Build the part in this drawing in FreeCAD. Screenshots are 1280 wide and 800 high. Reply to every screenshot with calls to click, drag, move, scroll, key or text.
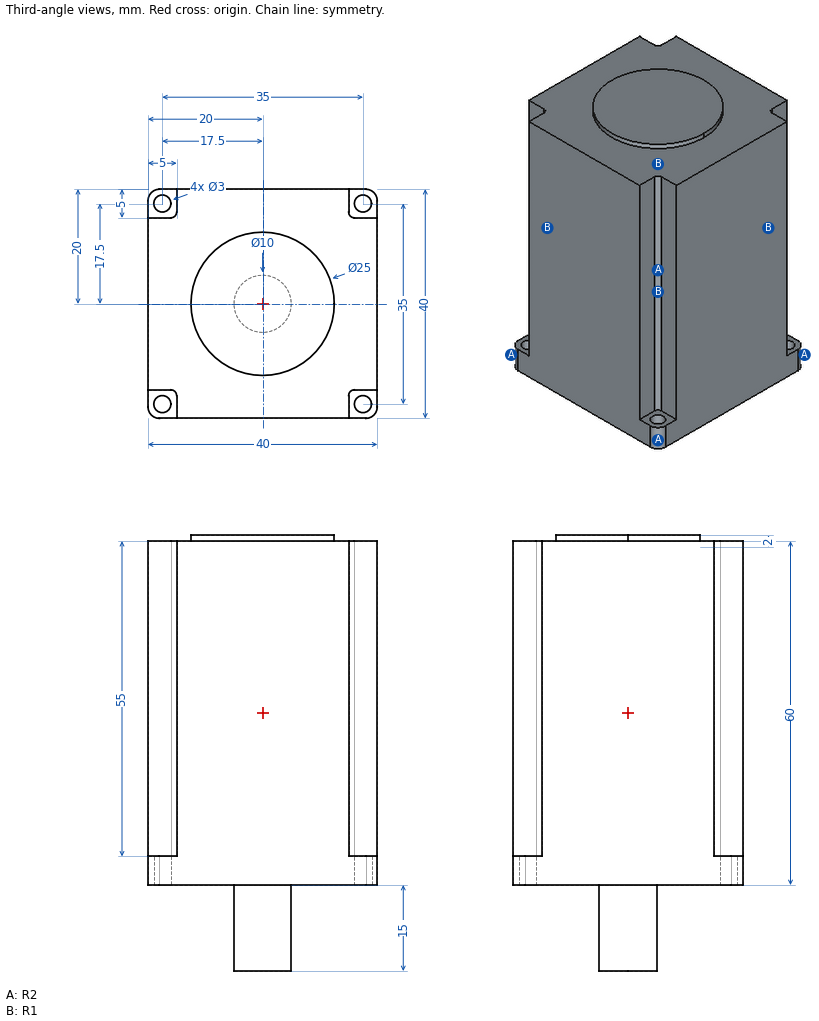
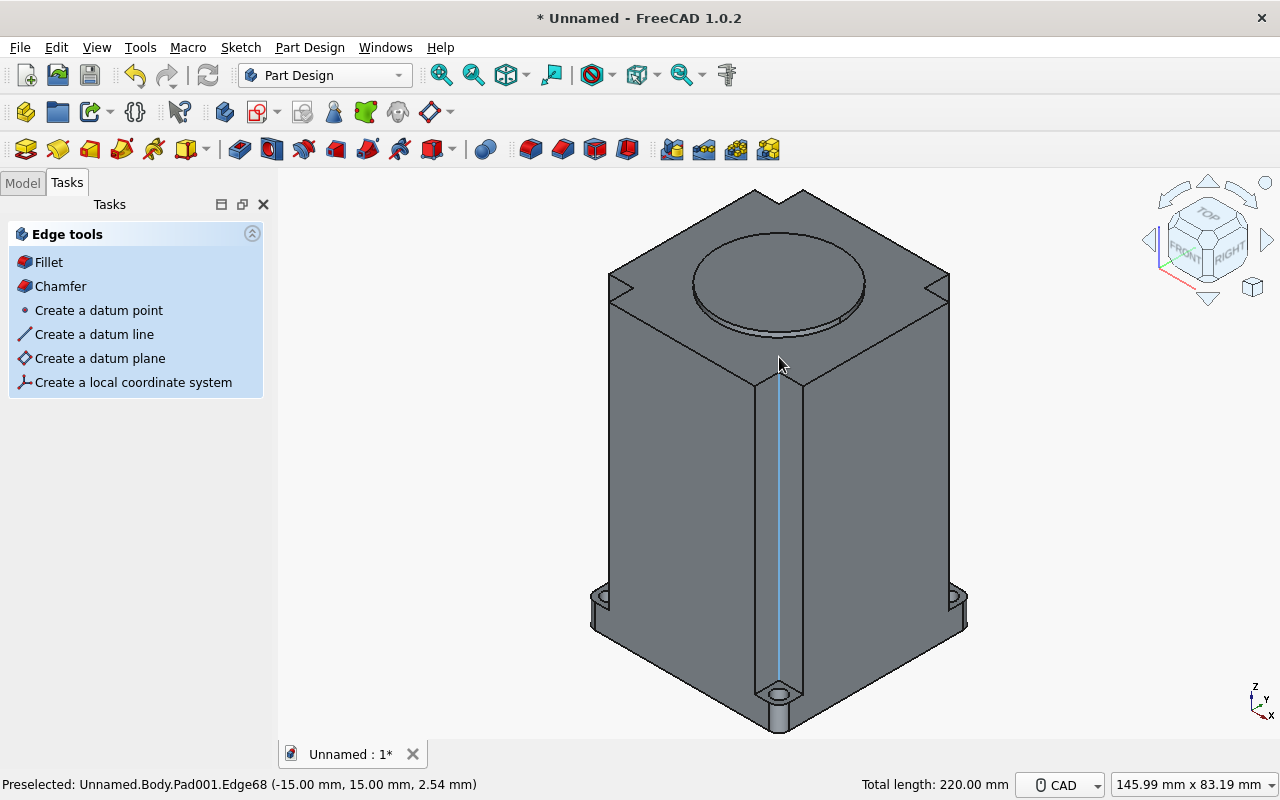
click(532, 150)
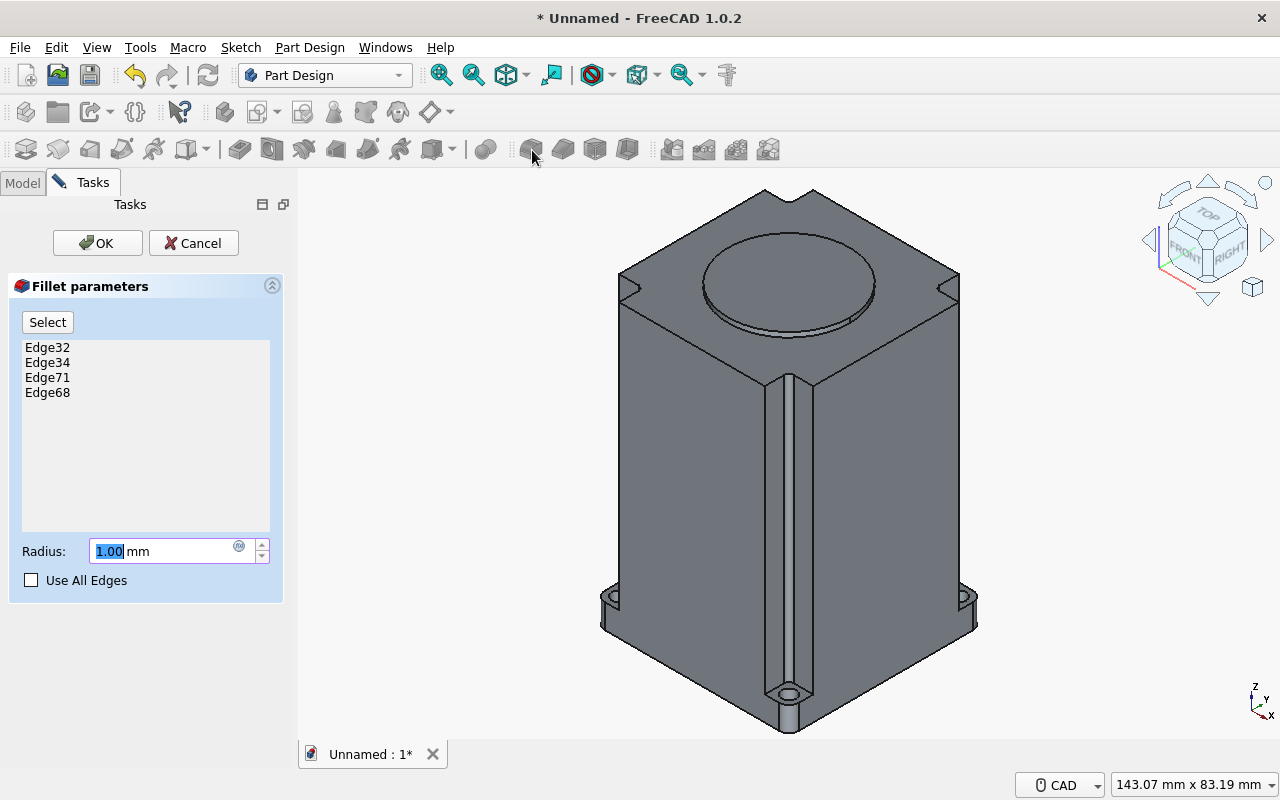
text(1)
key(Tab)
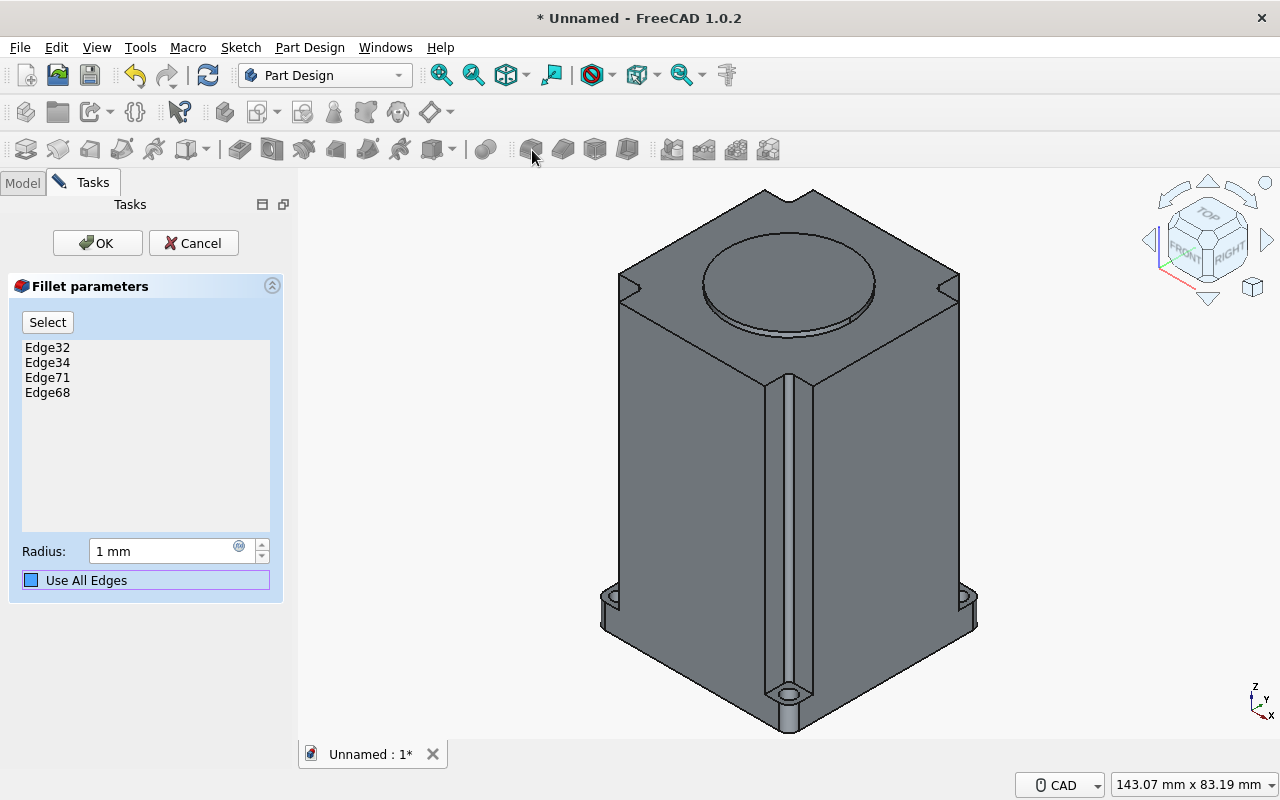
click(98, 243)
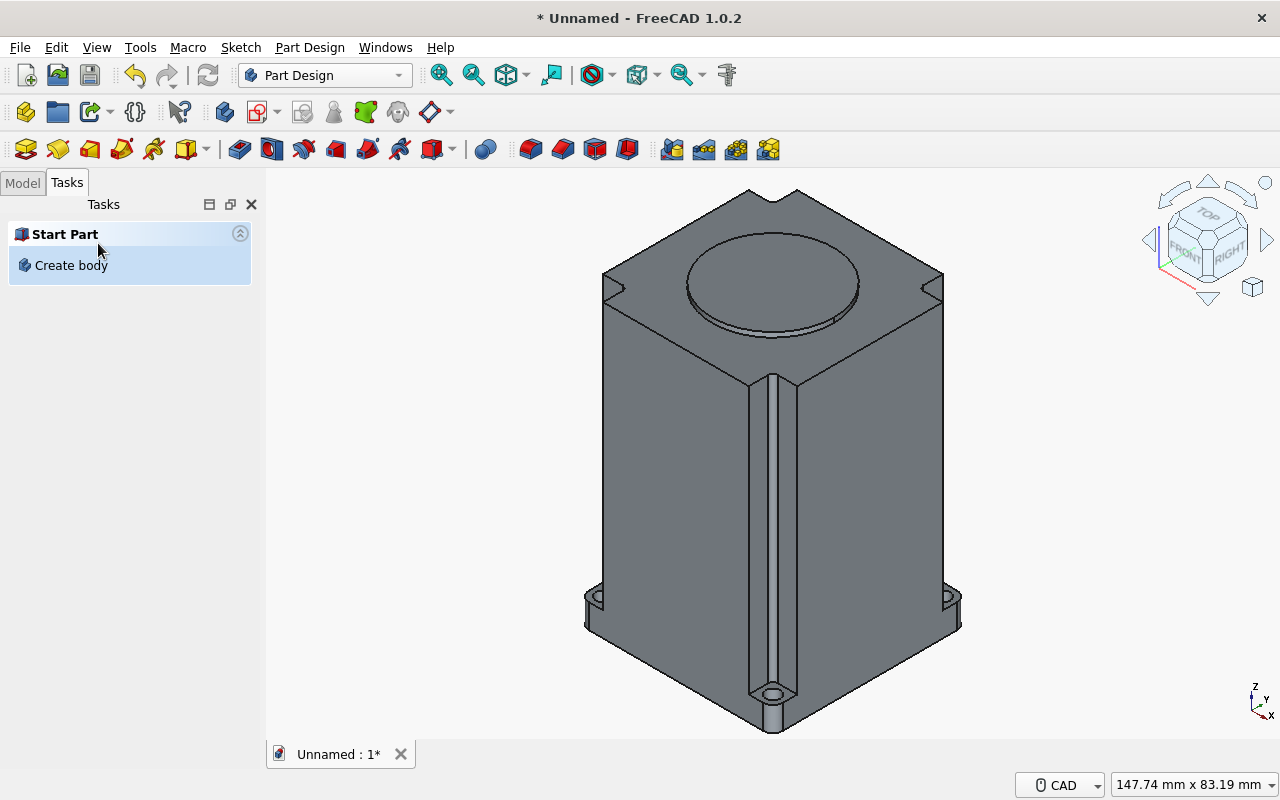
key(5)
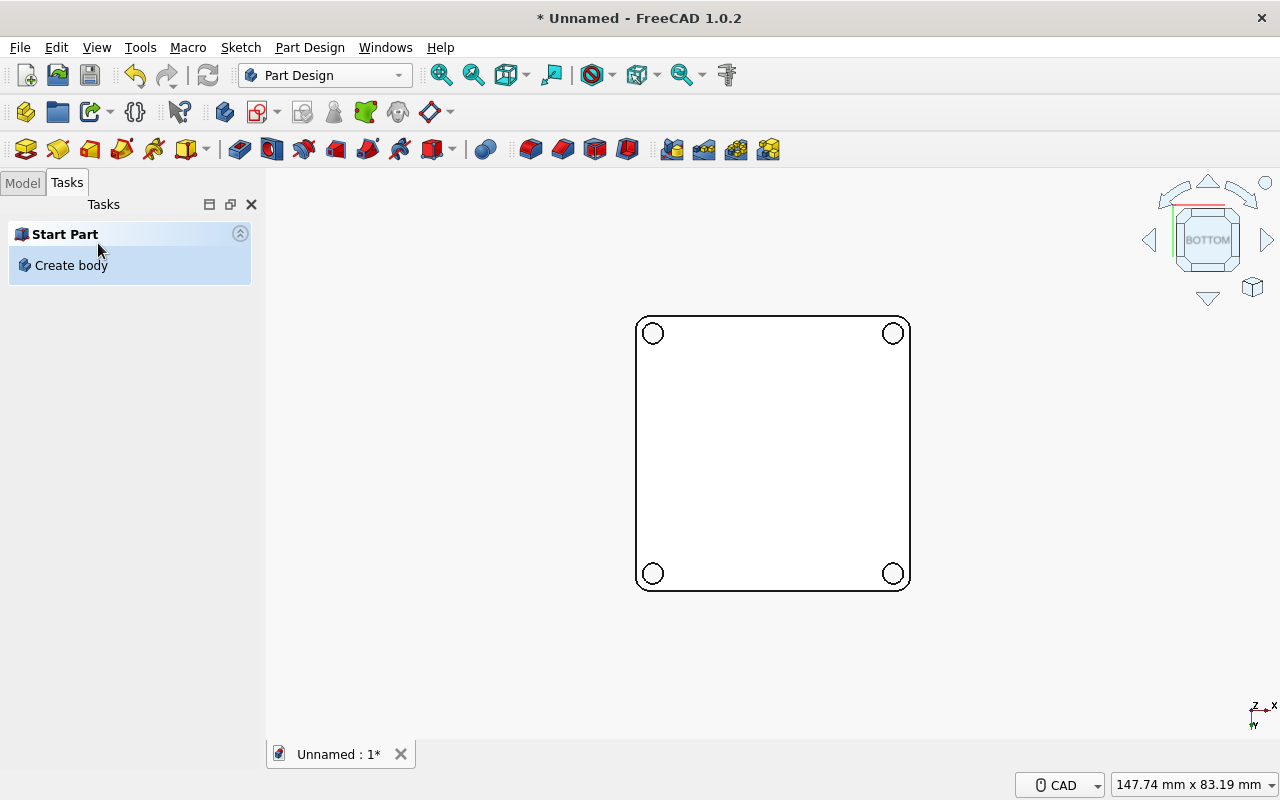
click(773, 452)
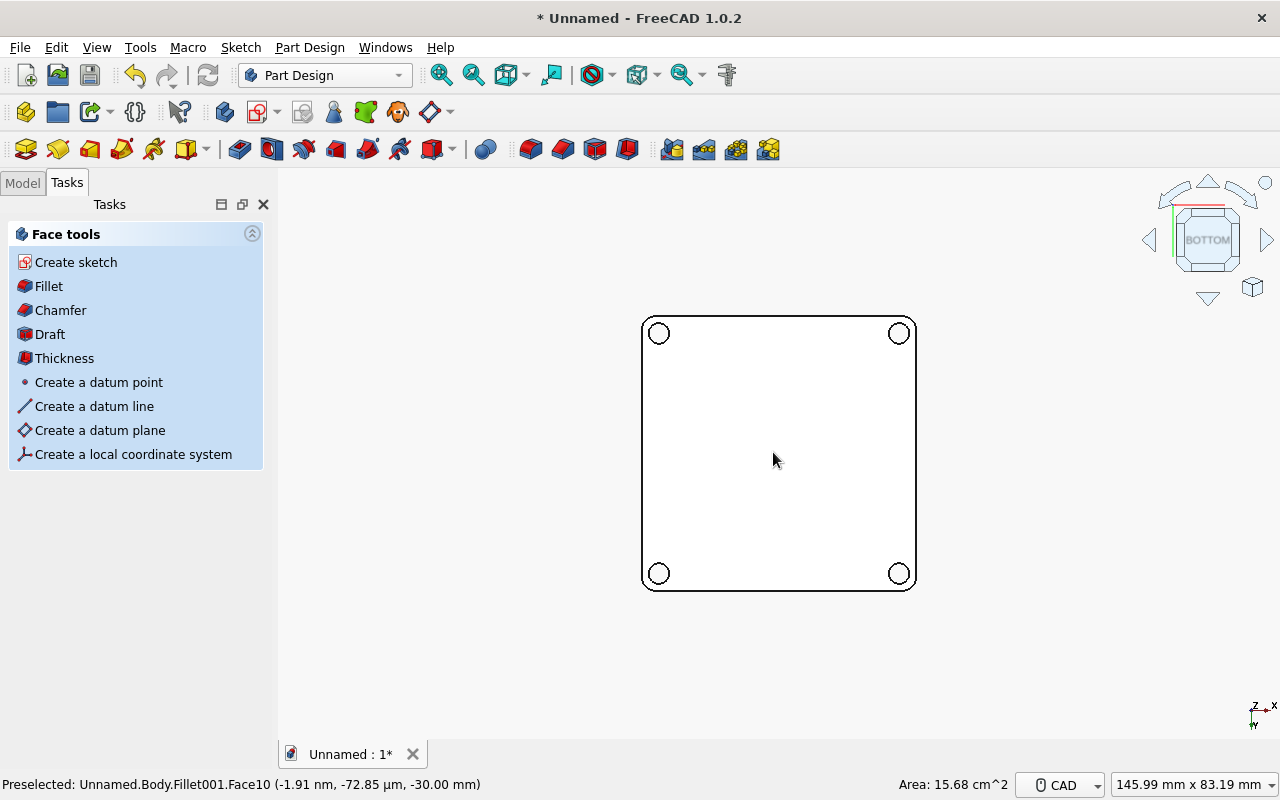
click(258, 112)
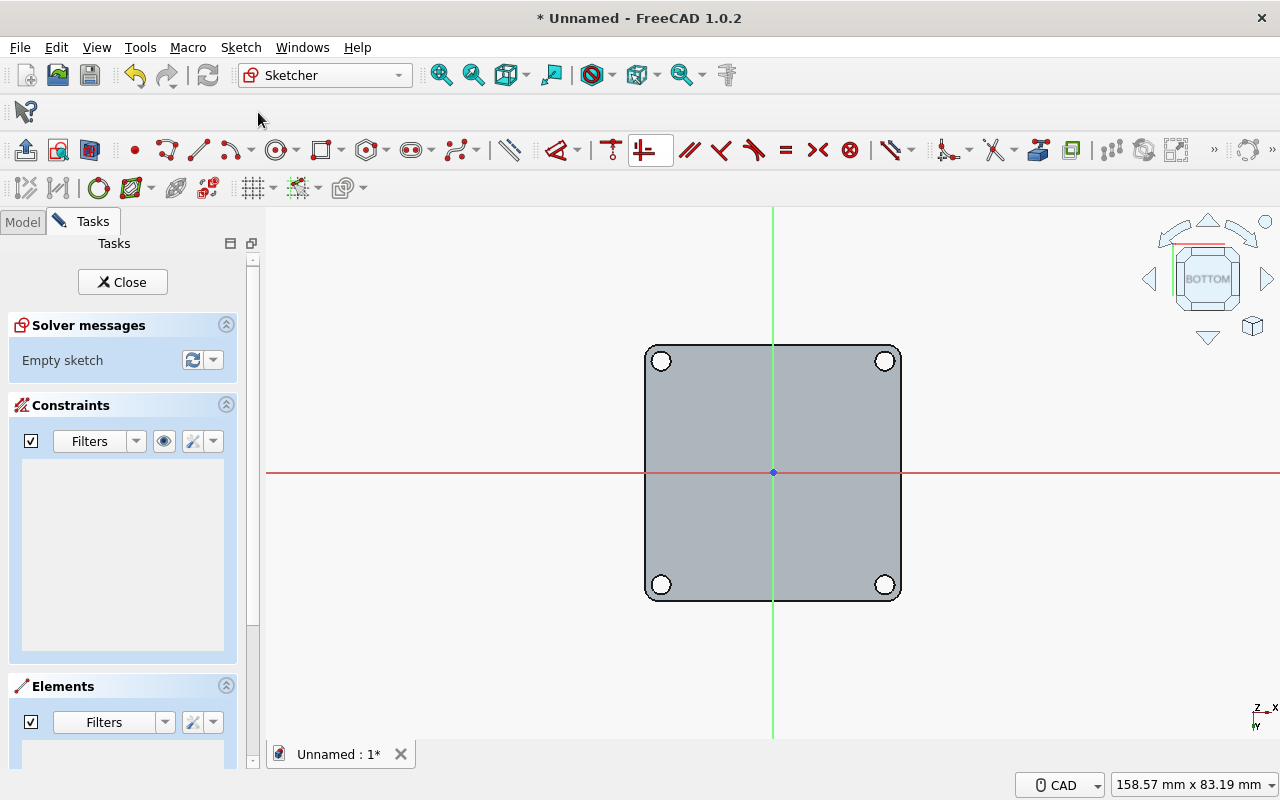
scroll(790, 473, up, 8)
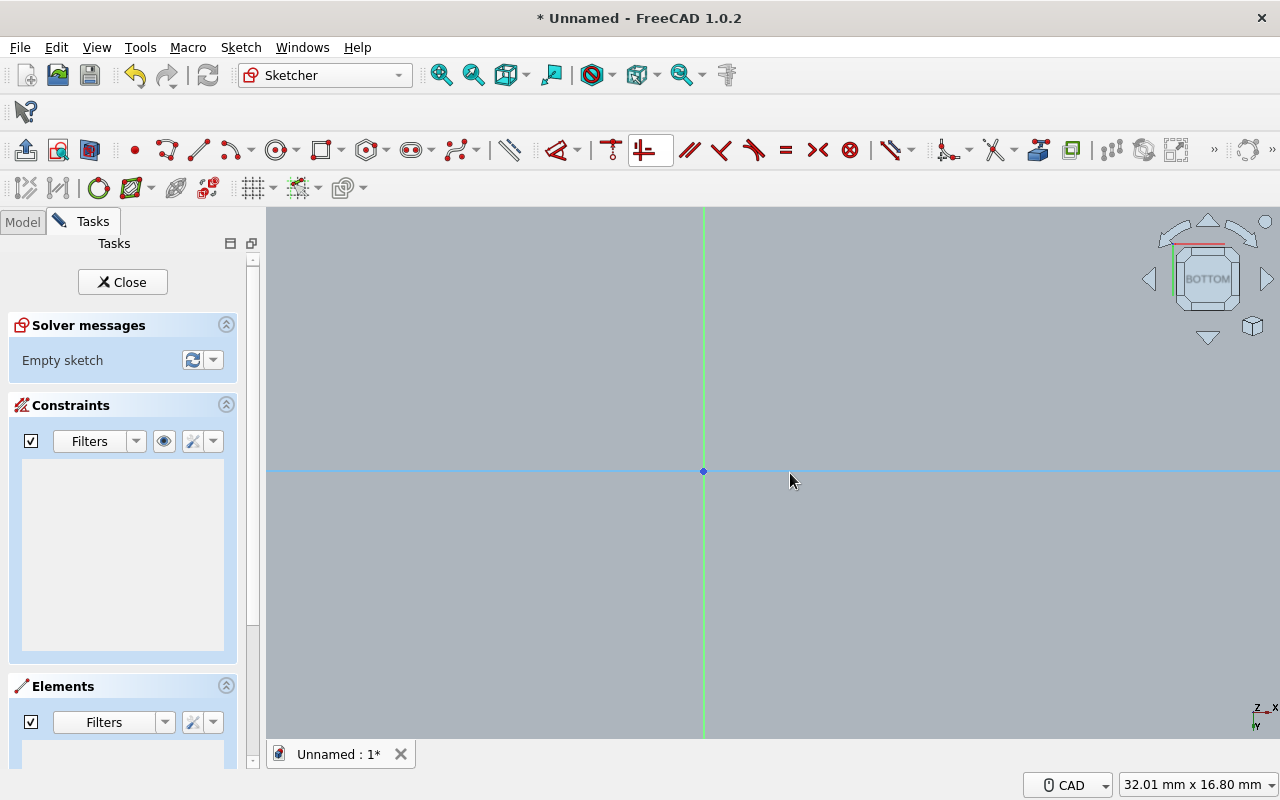
click(276, 150)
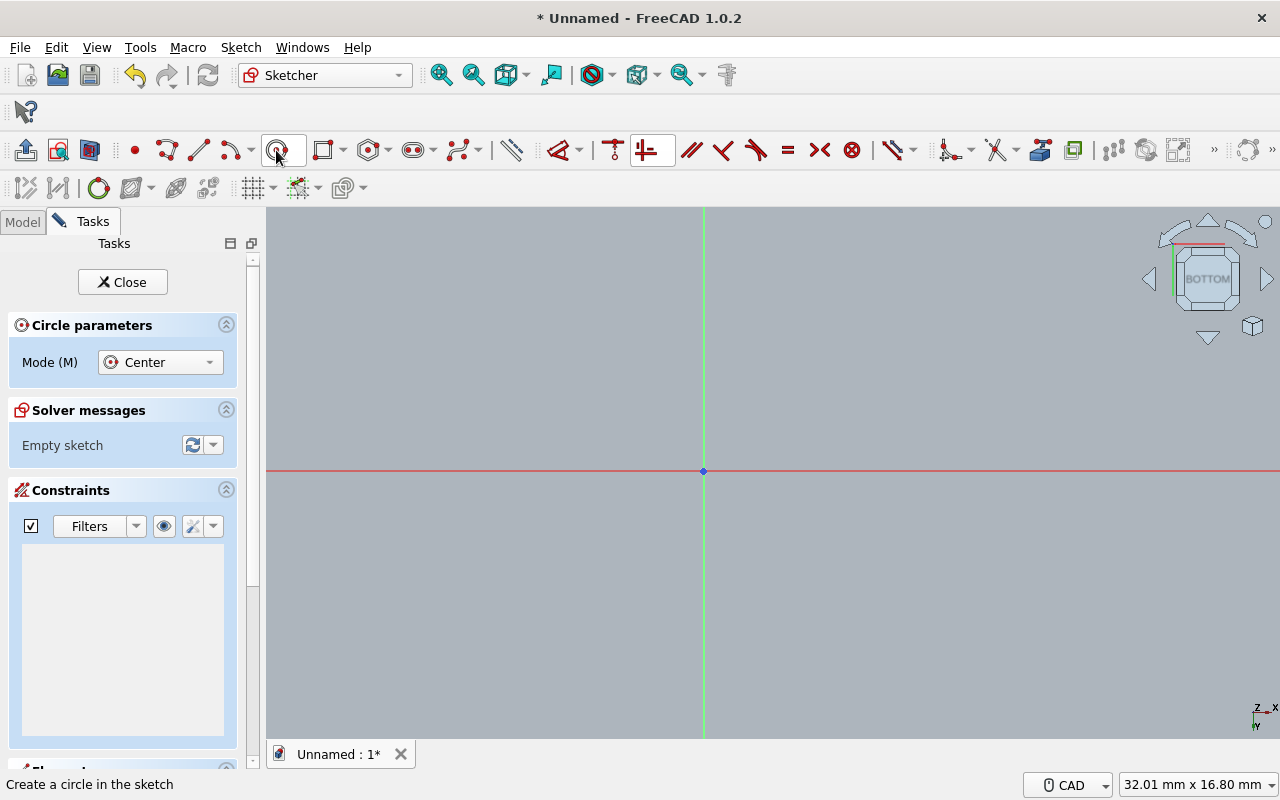
click(704, 471)
click(816, 359)
key(Escape)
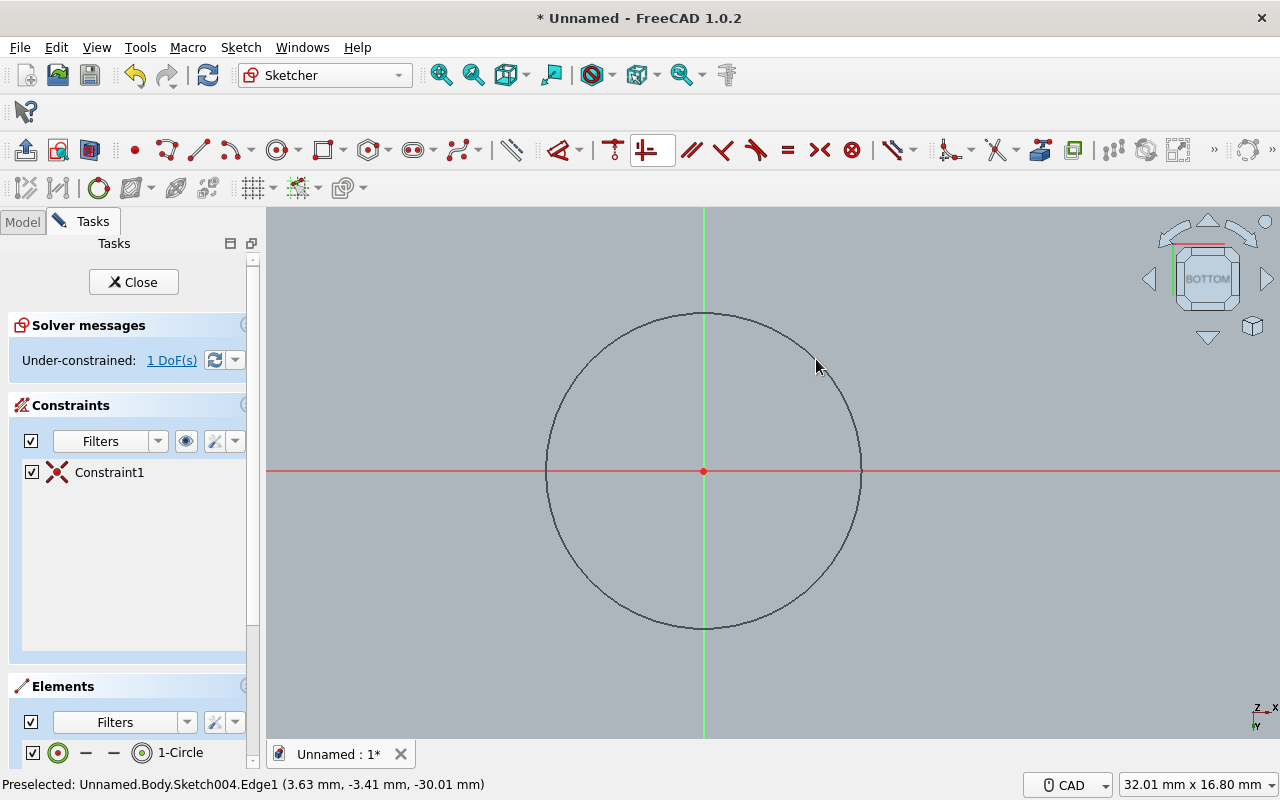
click(558, 150)